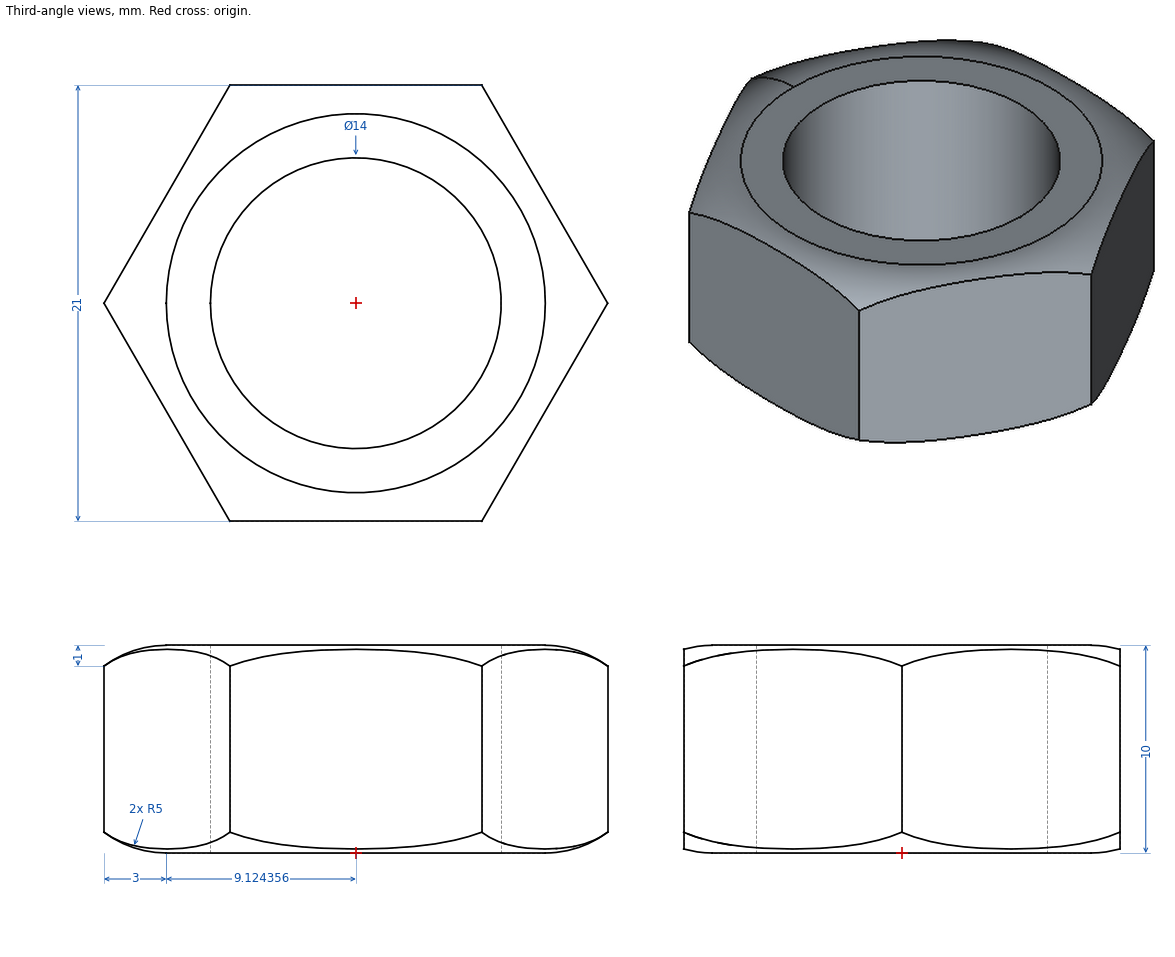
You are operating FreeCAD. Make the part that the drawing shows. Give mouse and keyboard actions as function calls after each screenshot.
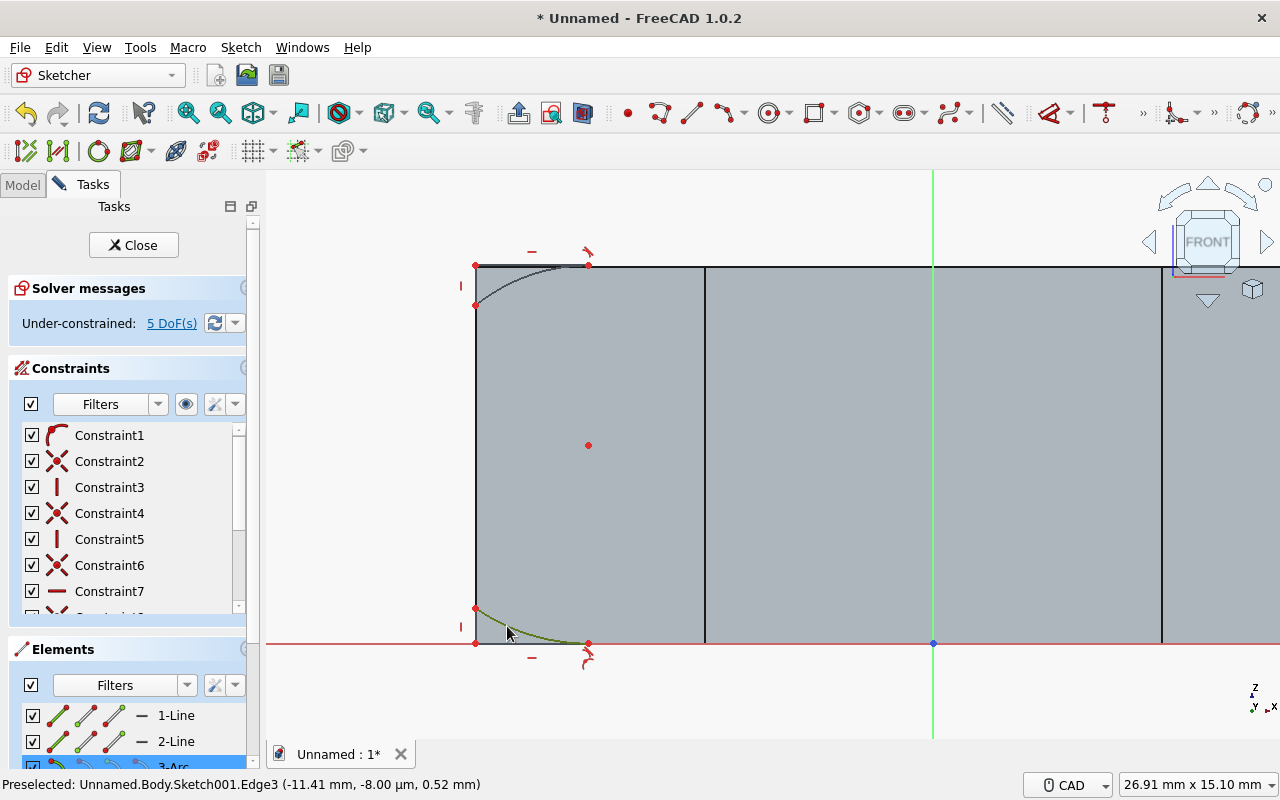
click(507, 285)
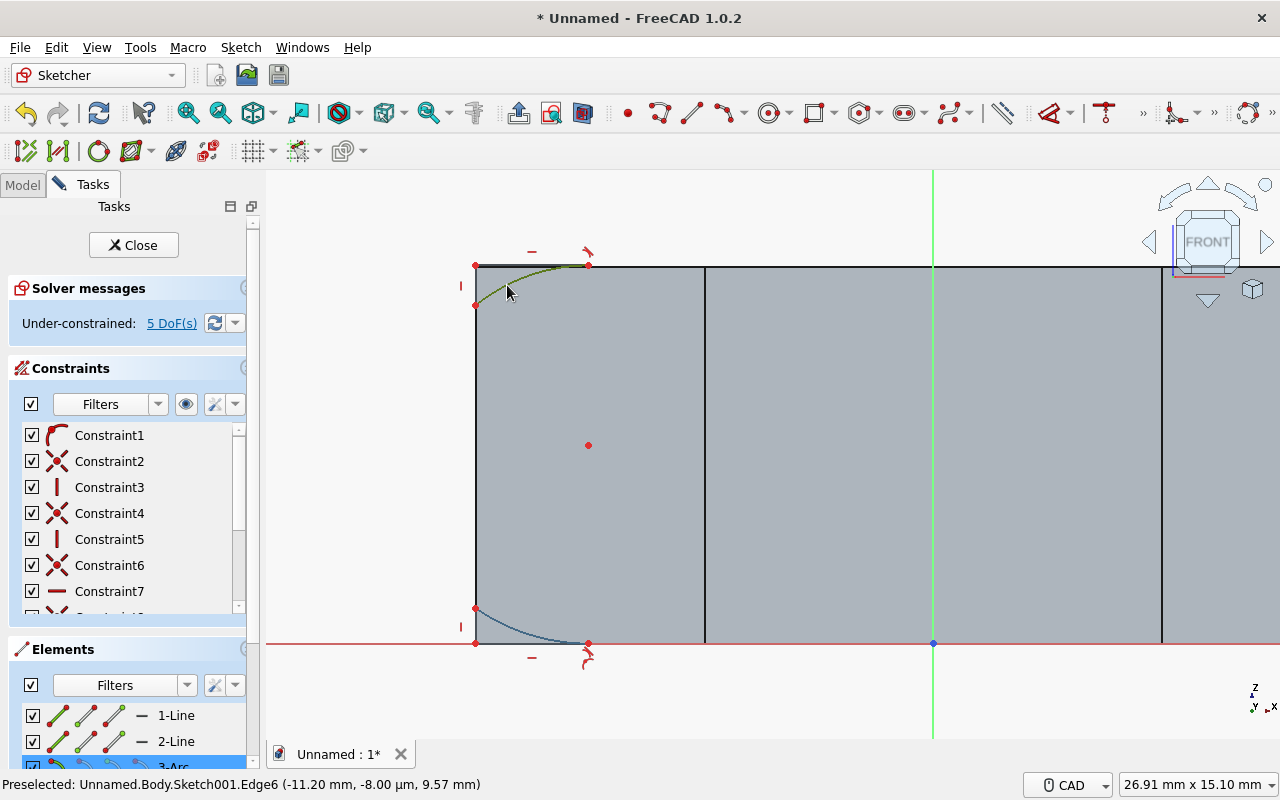
key(e)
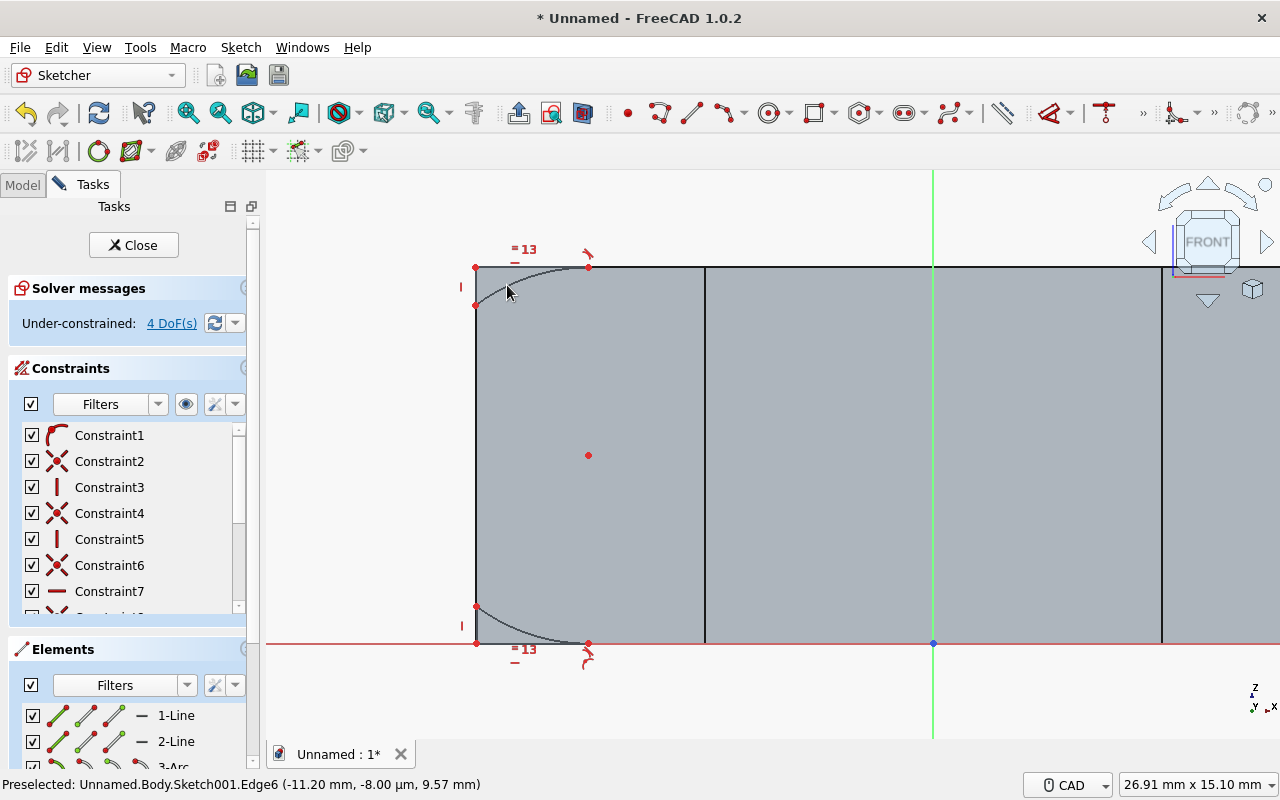
click(508, 625)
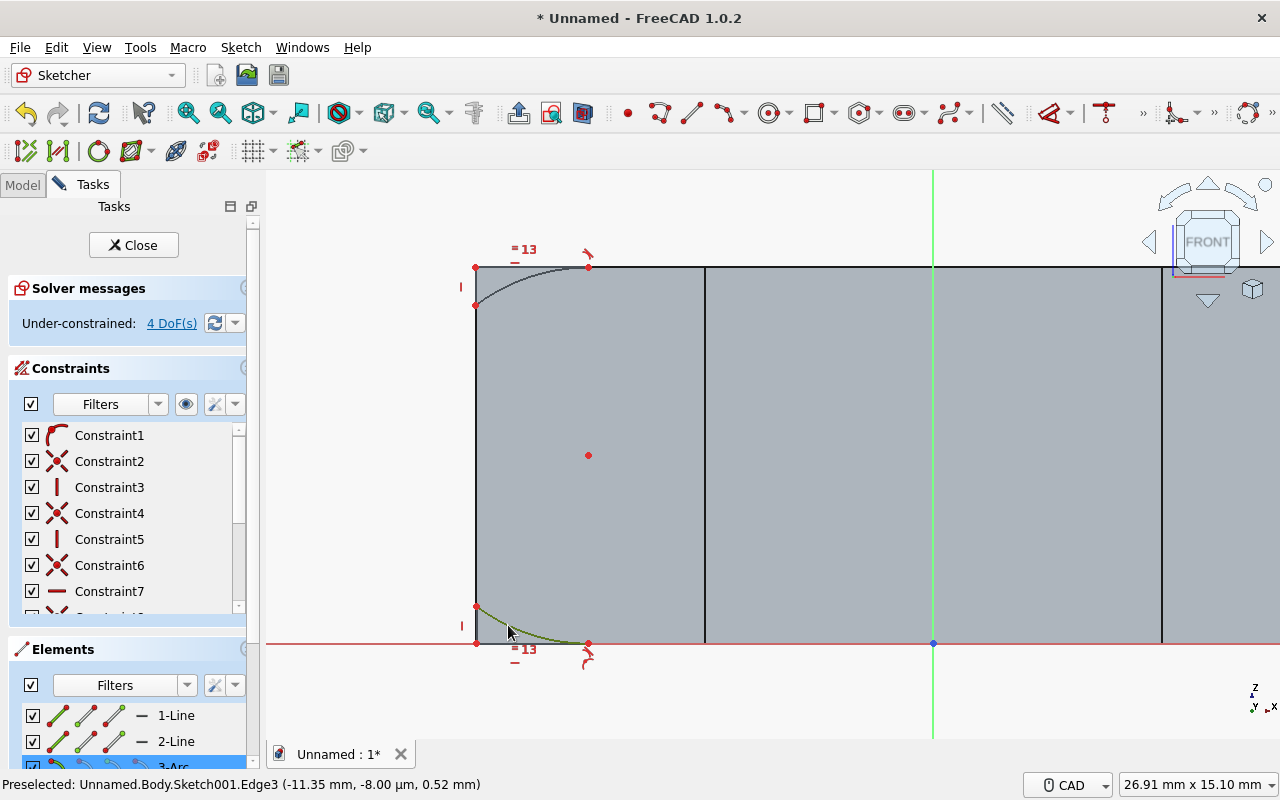
key(k)
key(r)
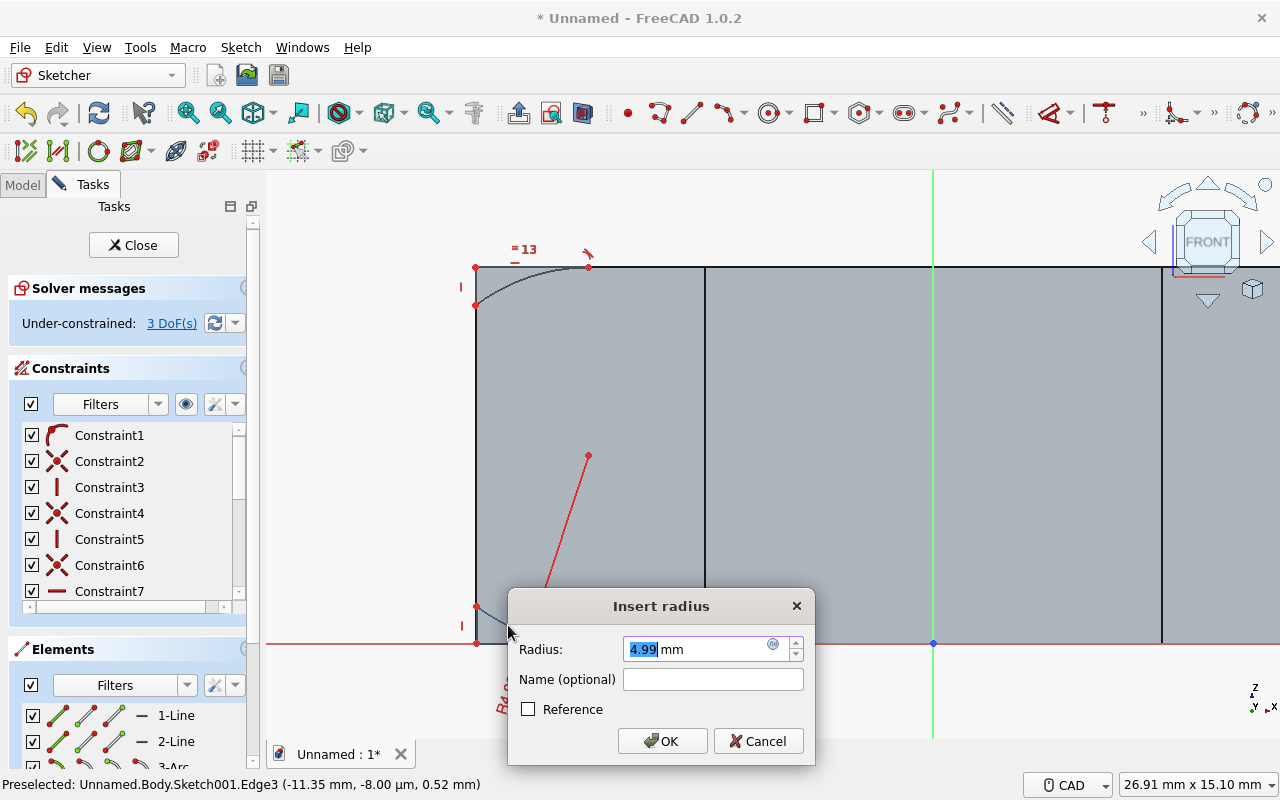
text(5)
key(Return)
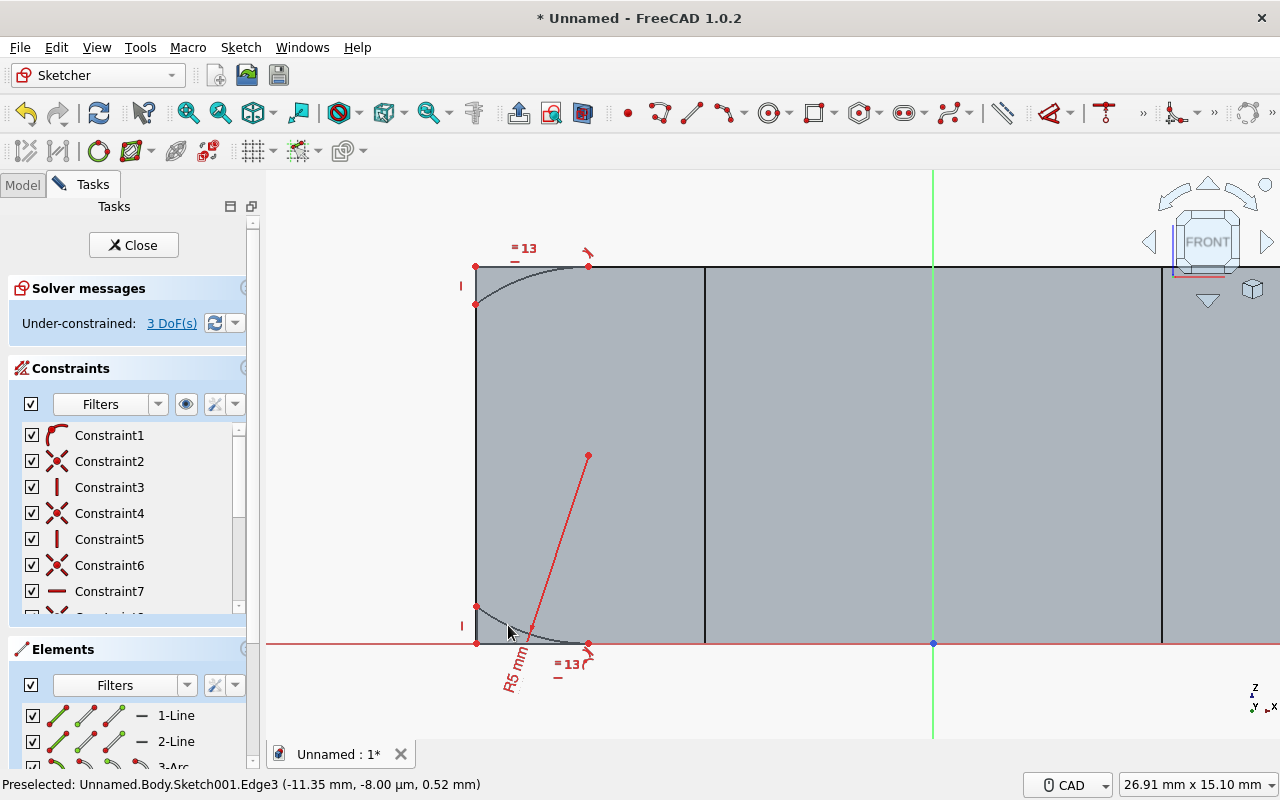
click(510, 644)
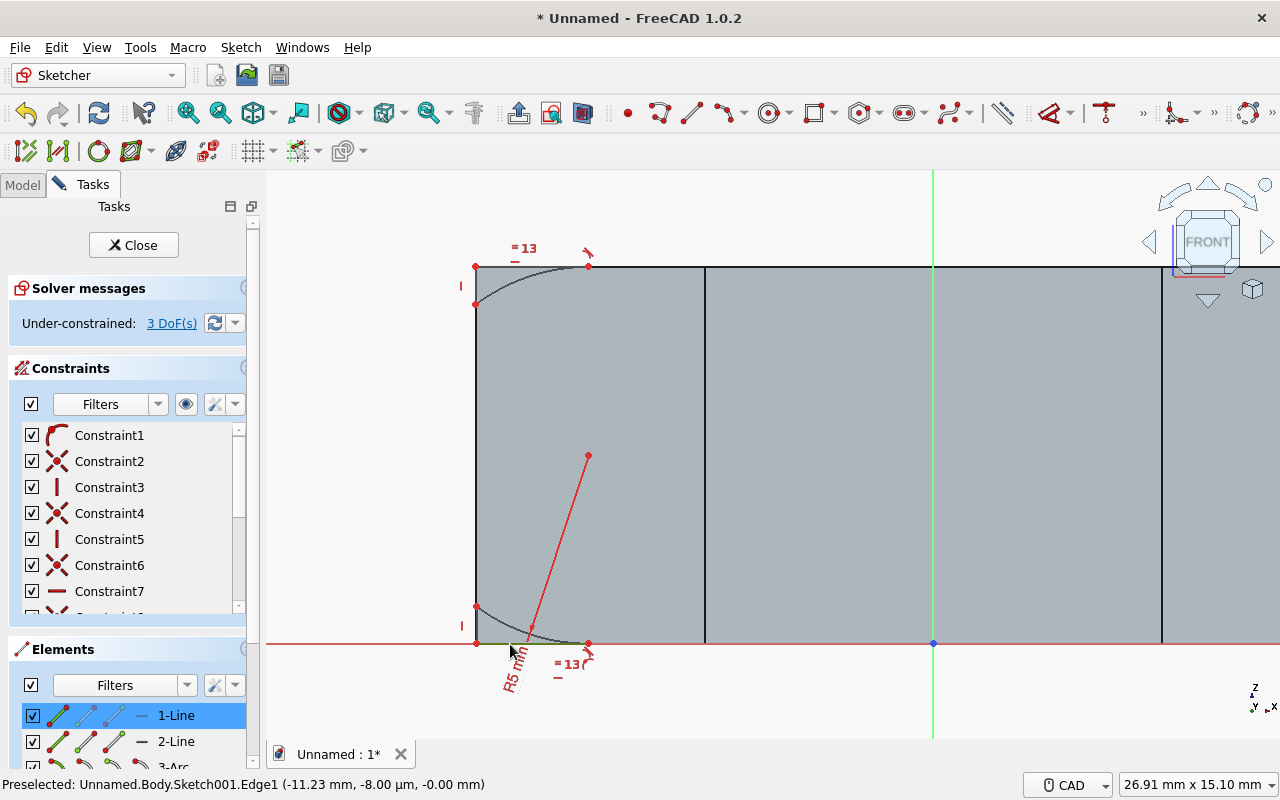
key(l)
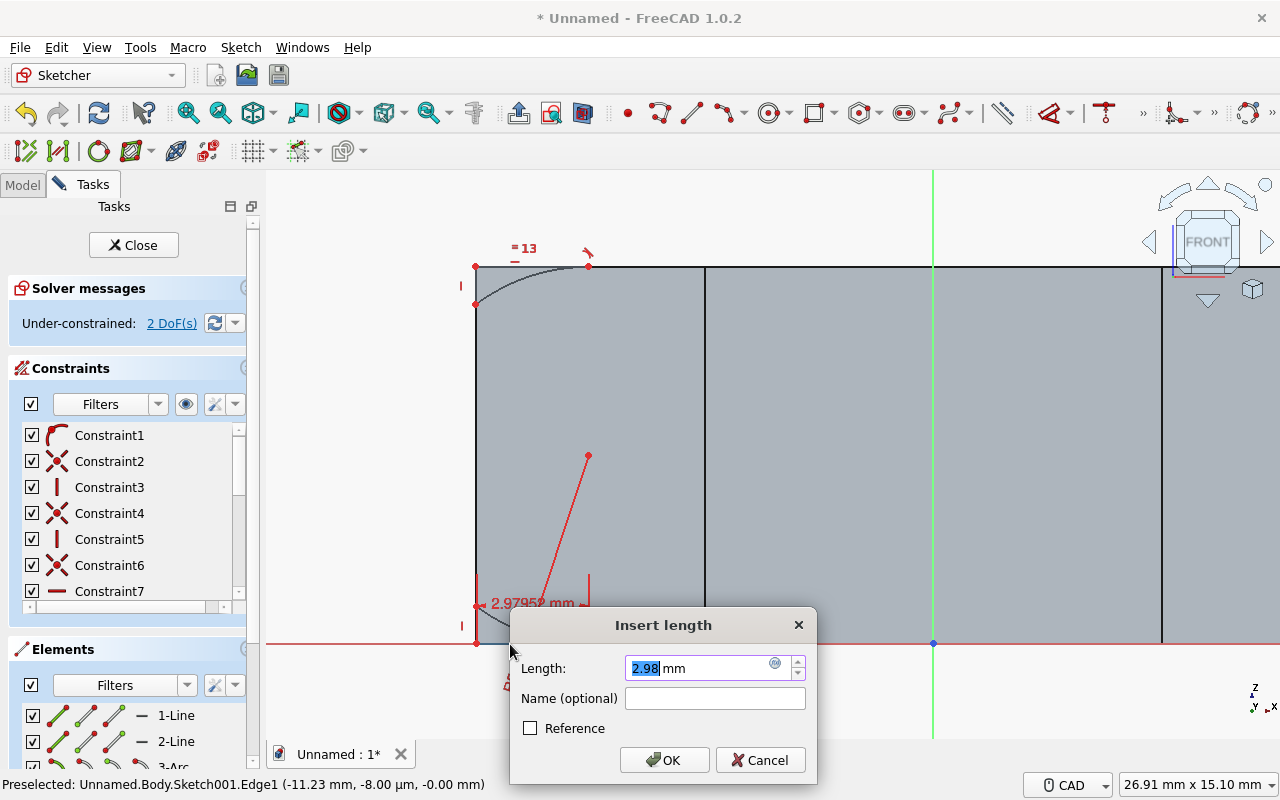
text(3)
key(Return)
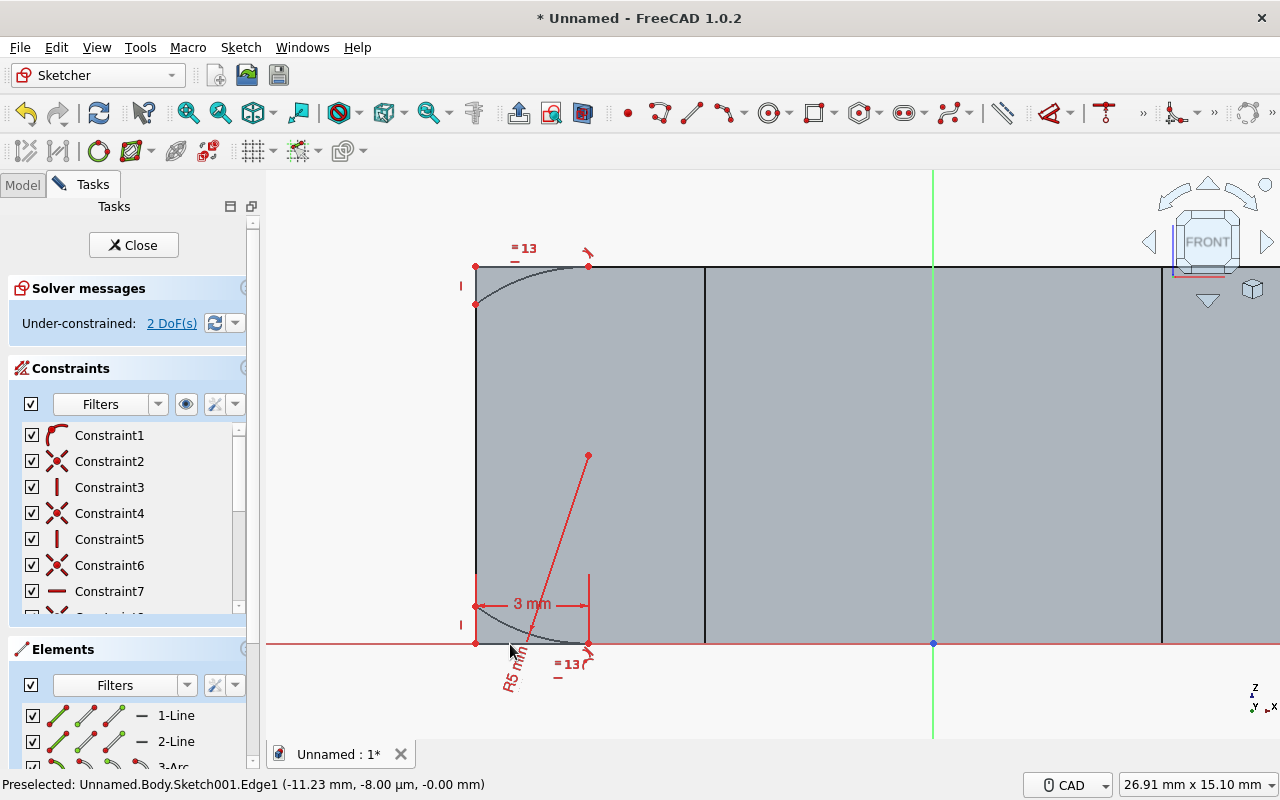
scroll(476, 293, up, 3)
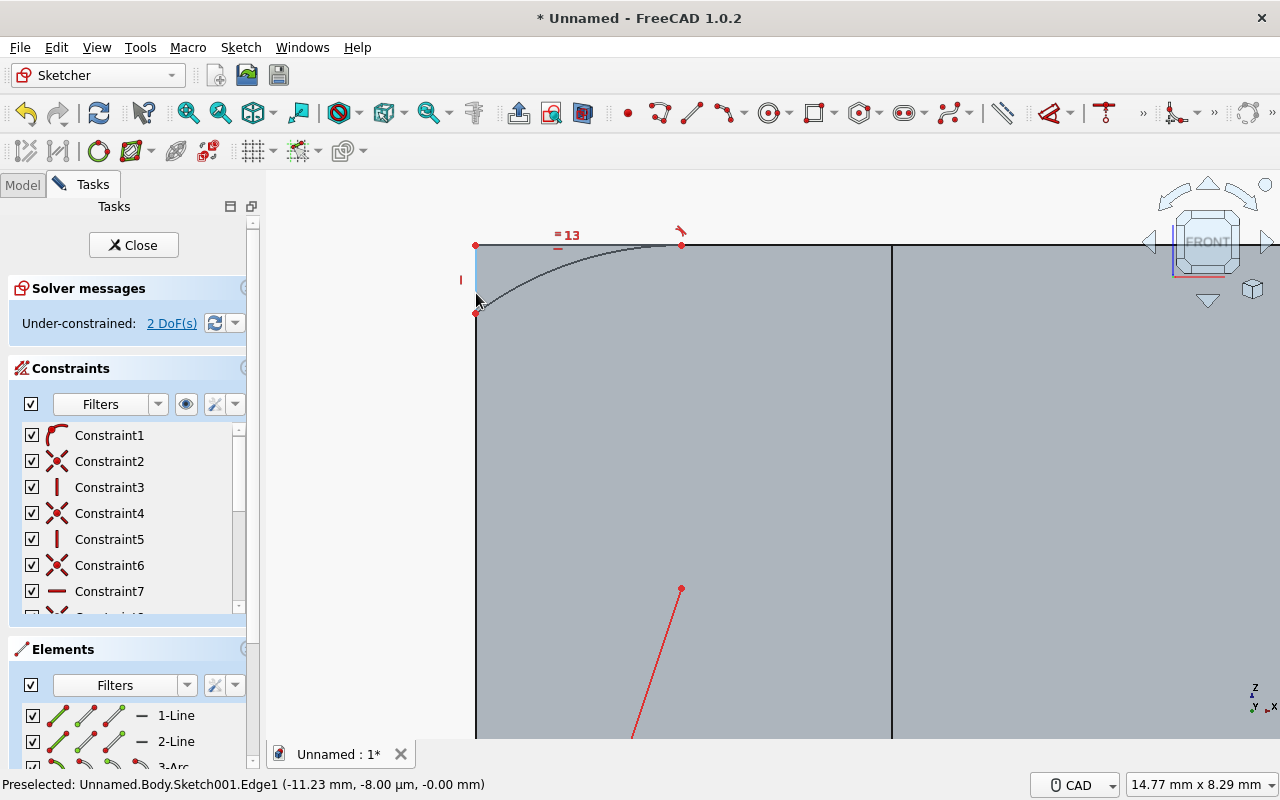
click(476, 293)